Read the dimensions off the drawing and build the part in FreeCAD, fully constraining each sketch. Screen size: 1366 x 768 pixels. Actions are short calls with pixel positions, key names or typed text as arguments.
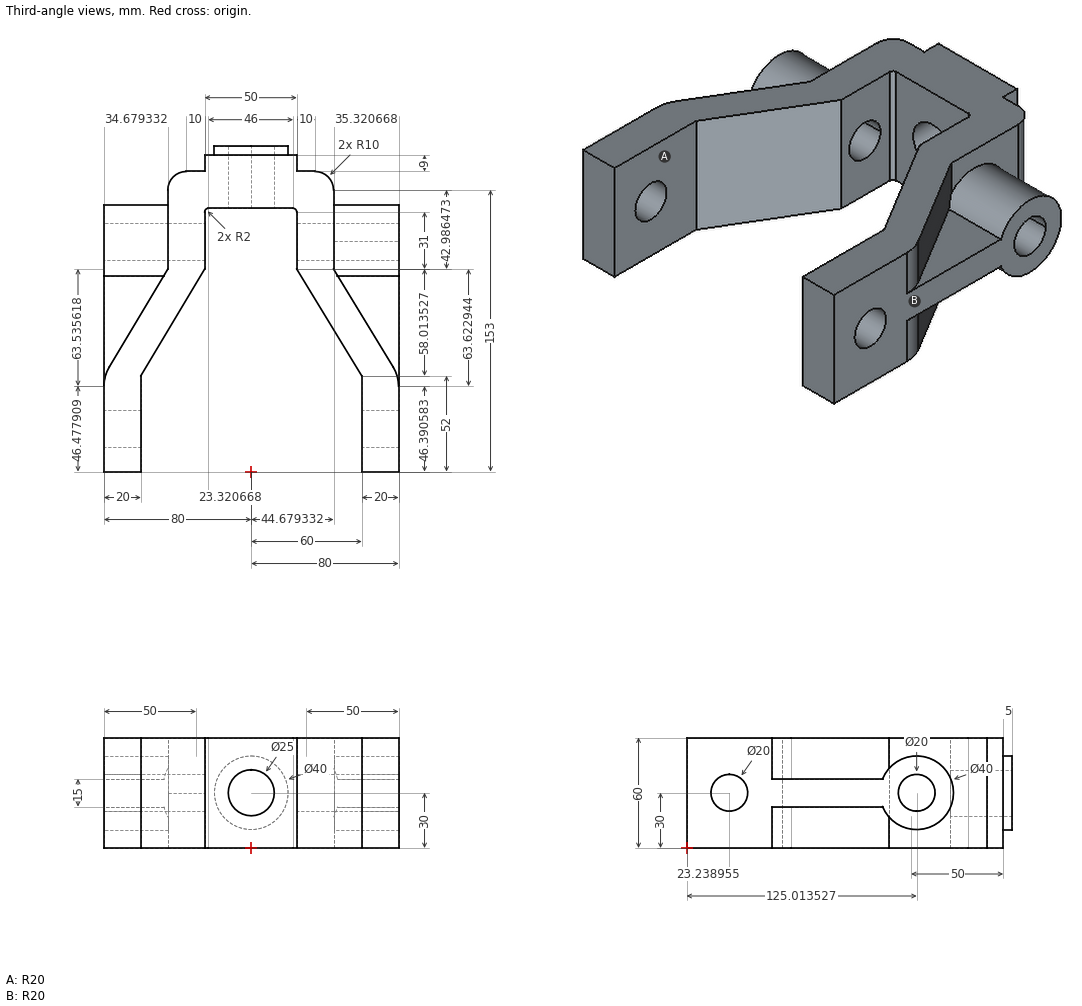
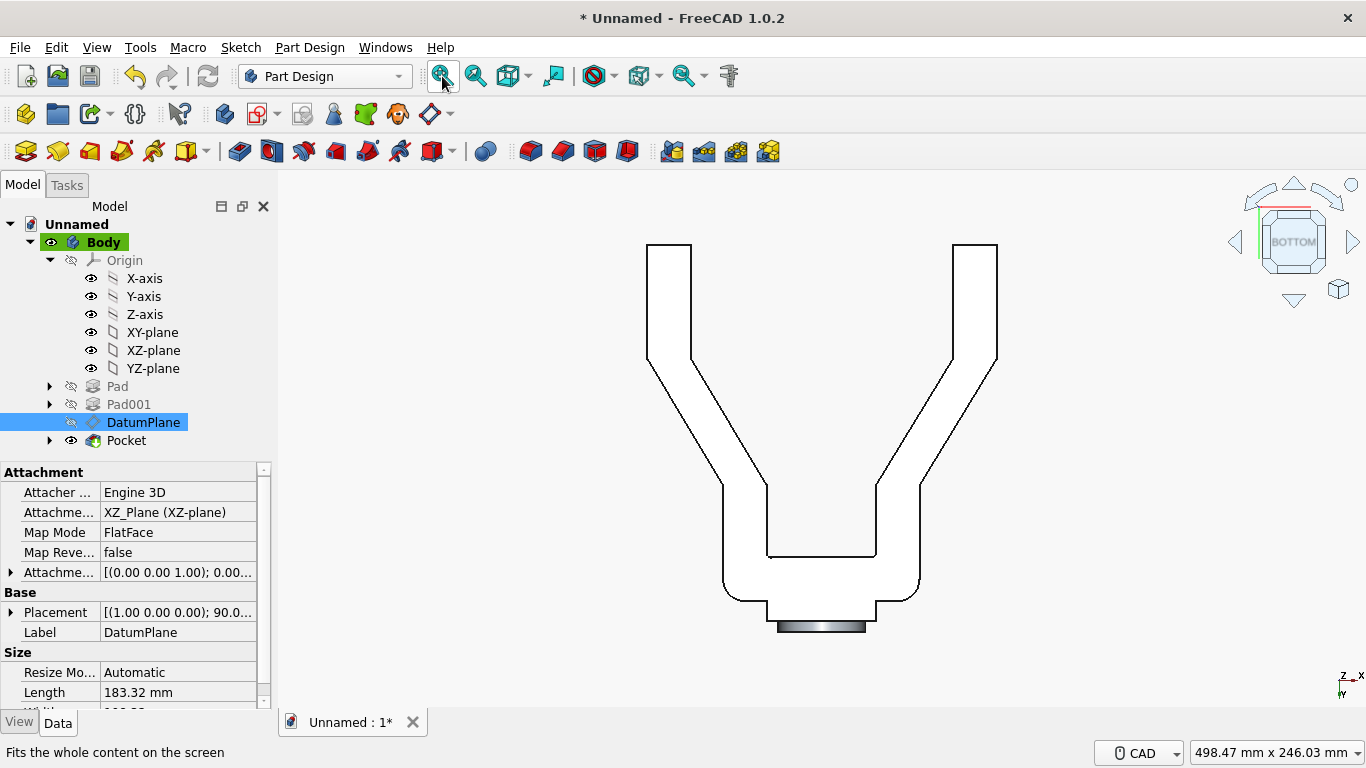
key(4)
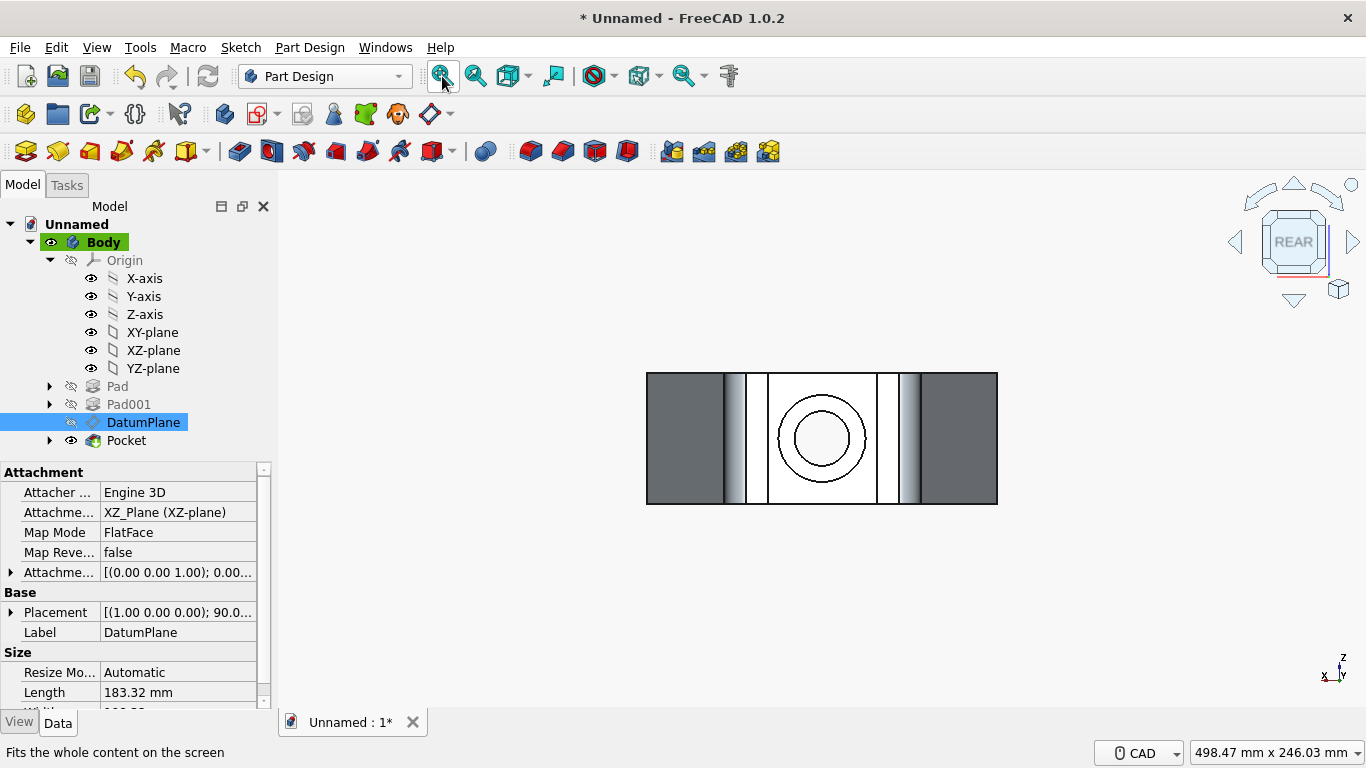
key(v)
key(f)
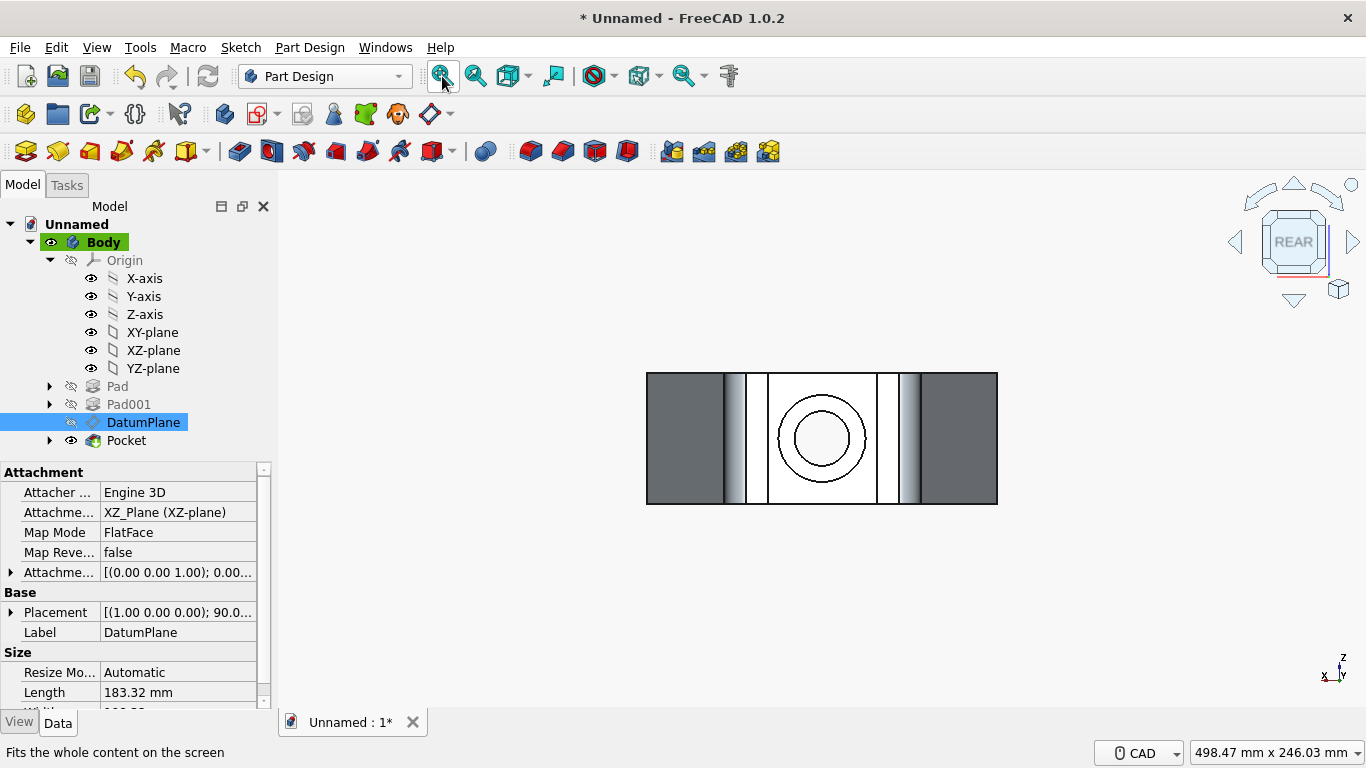
key(6)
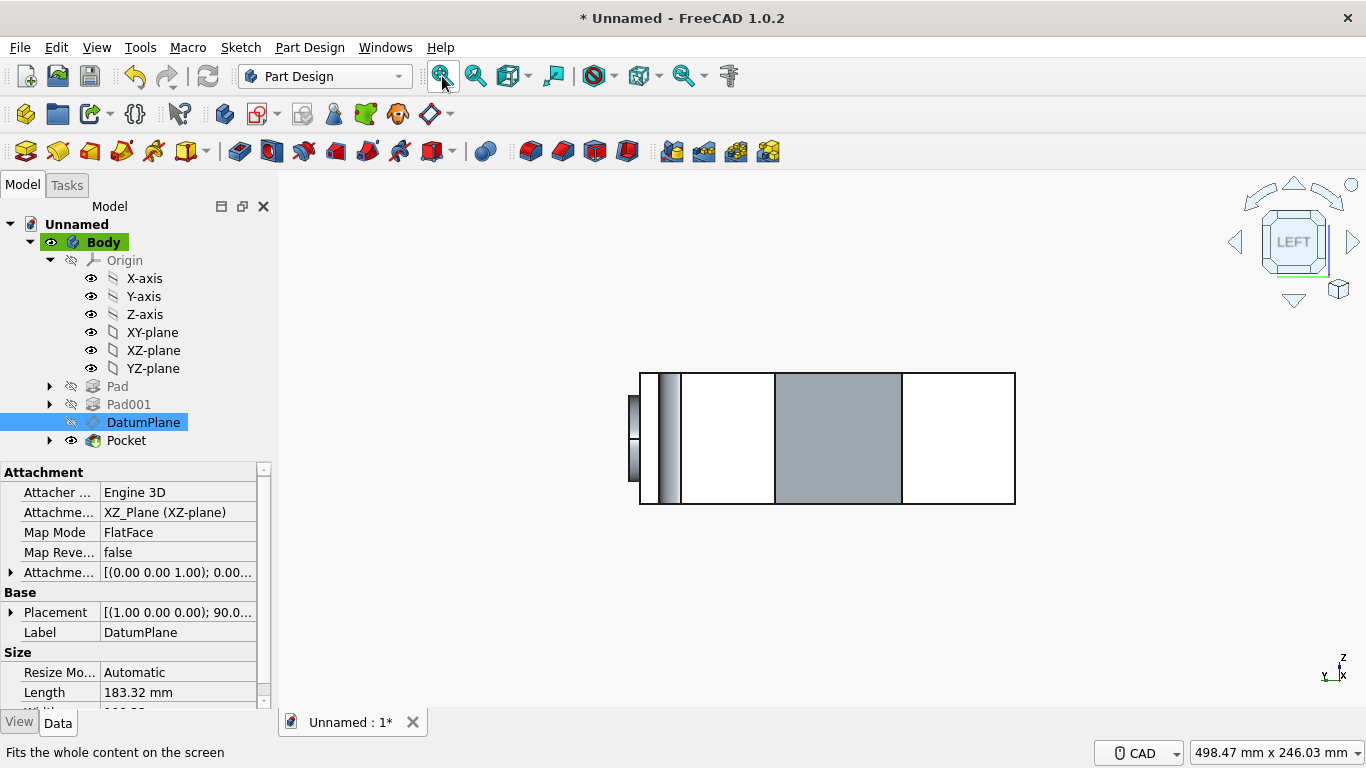
key(v)
key(f)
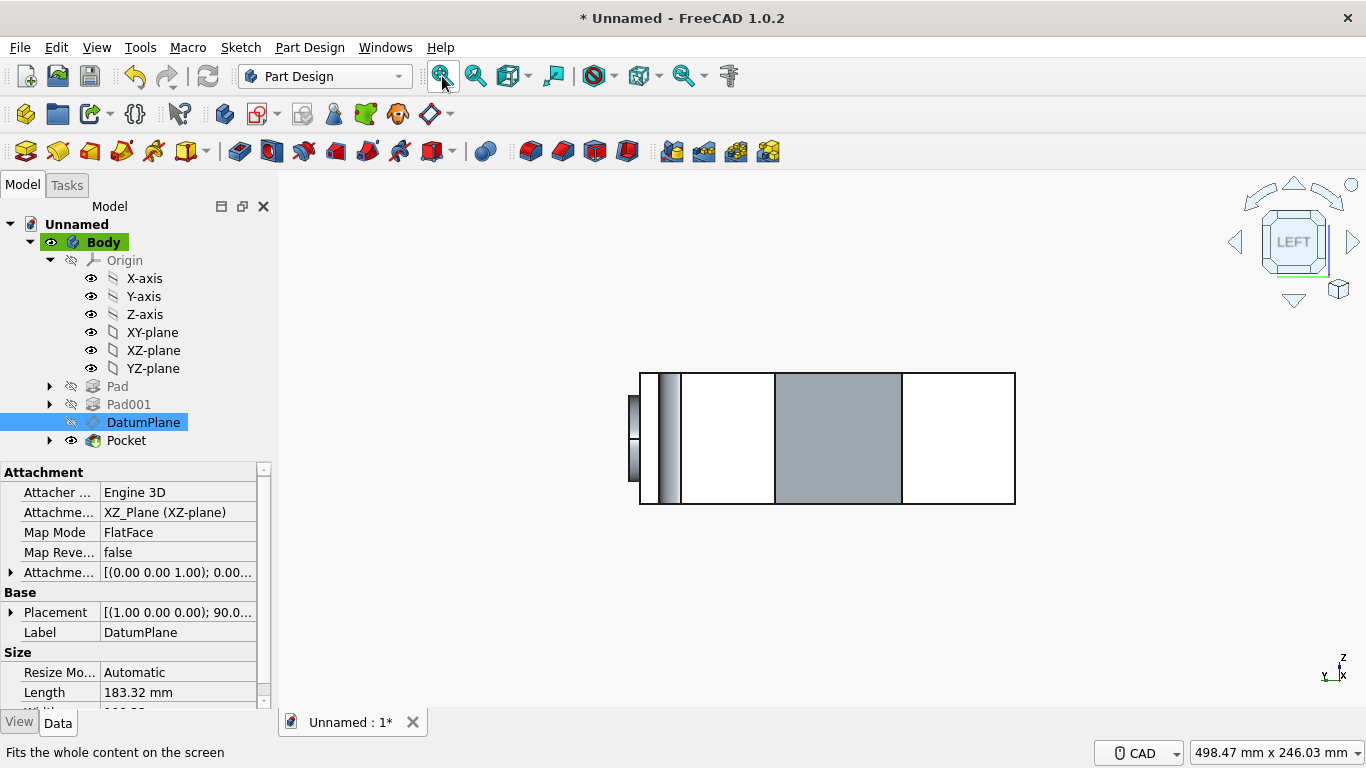
click(902, 437)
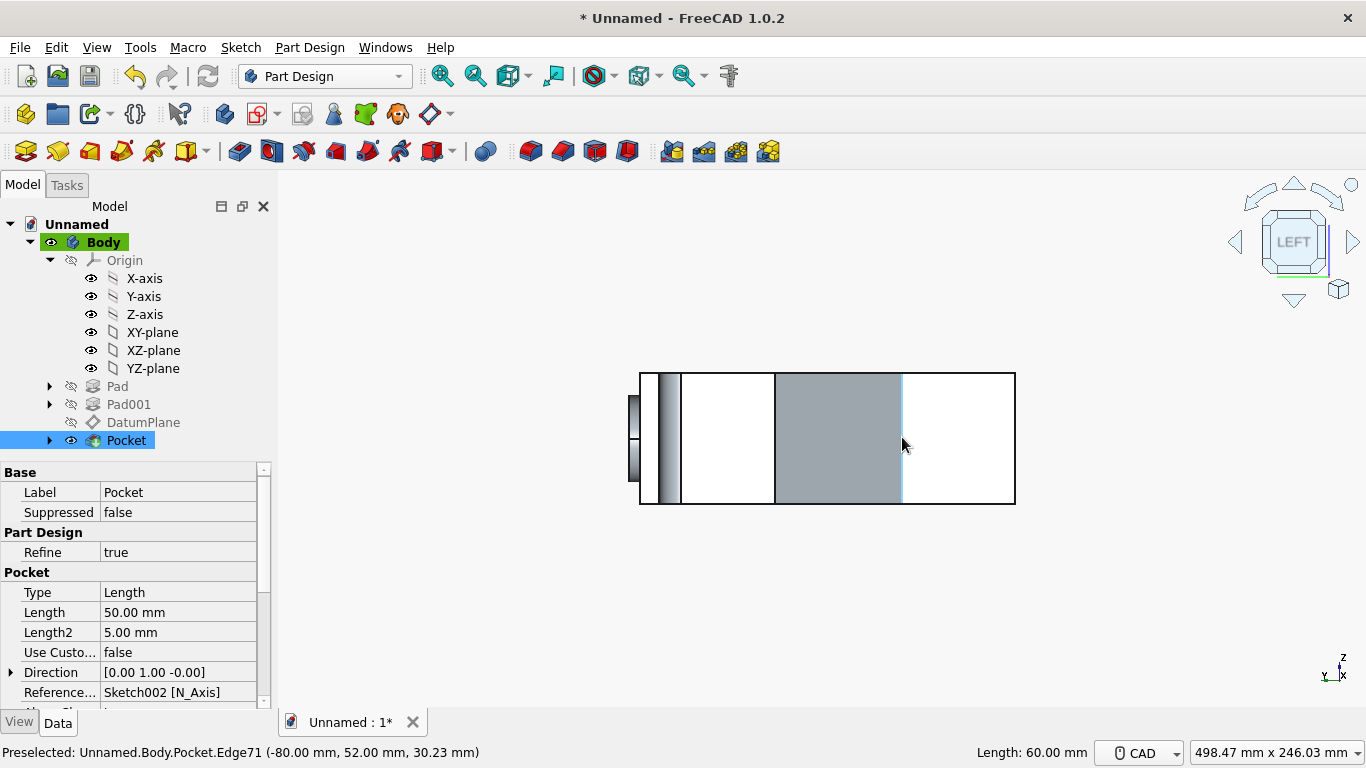
click(532, 152)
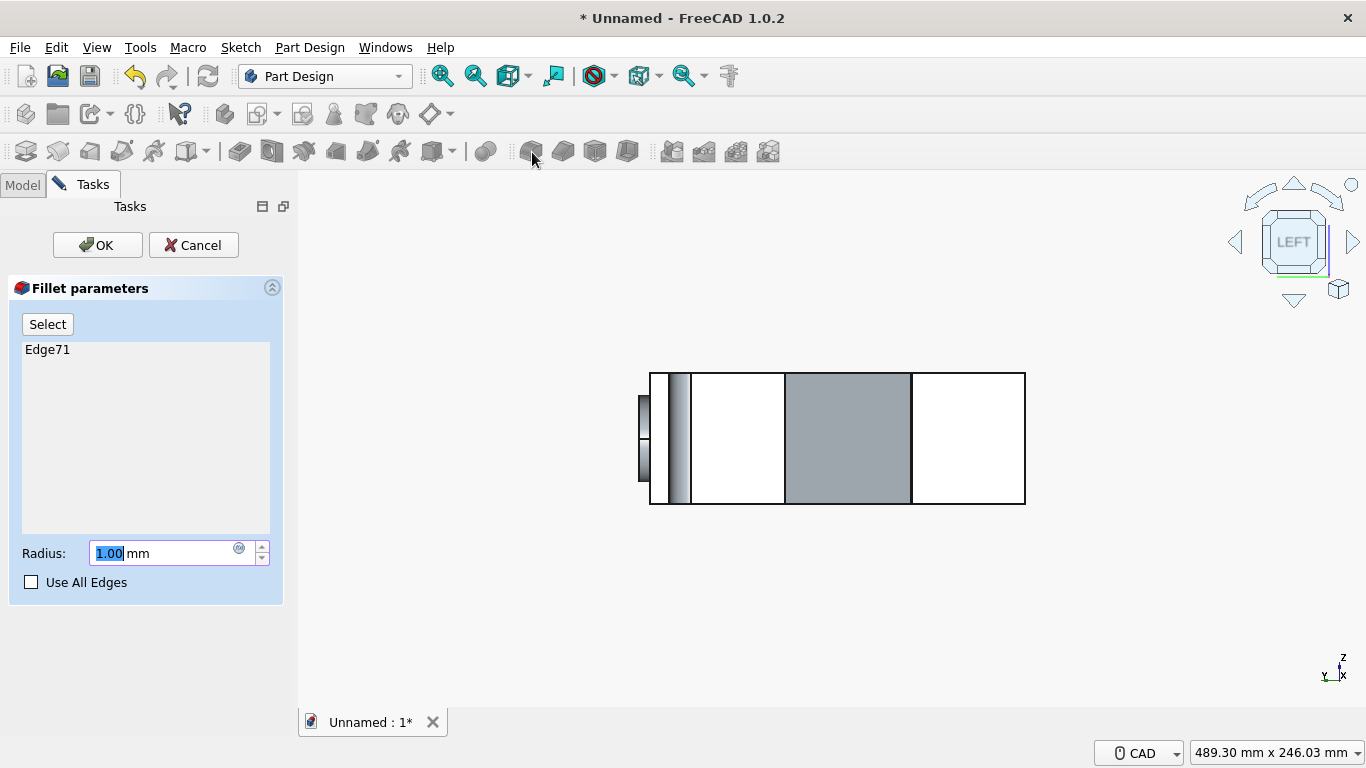
text(20)
key(Tab)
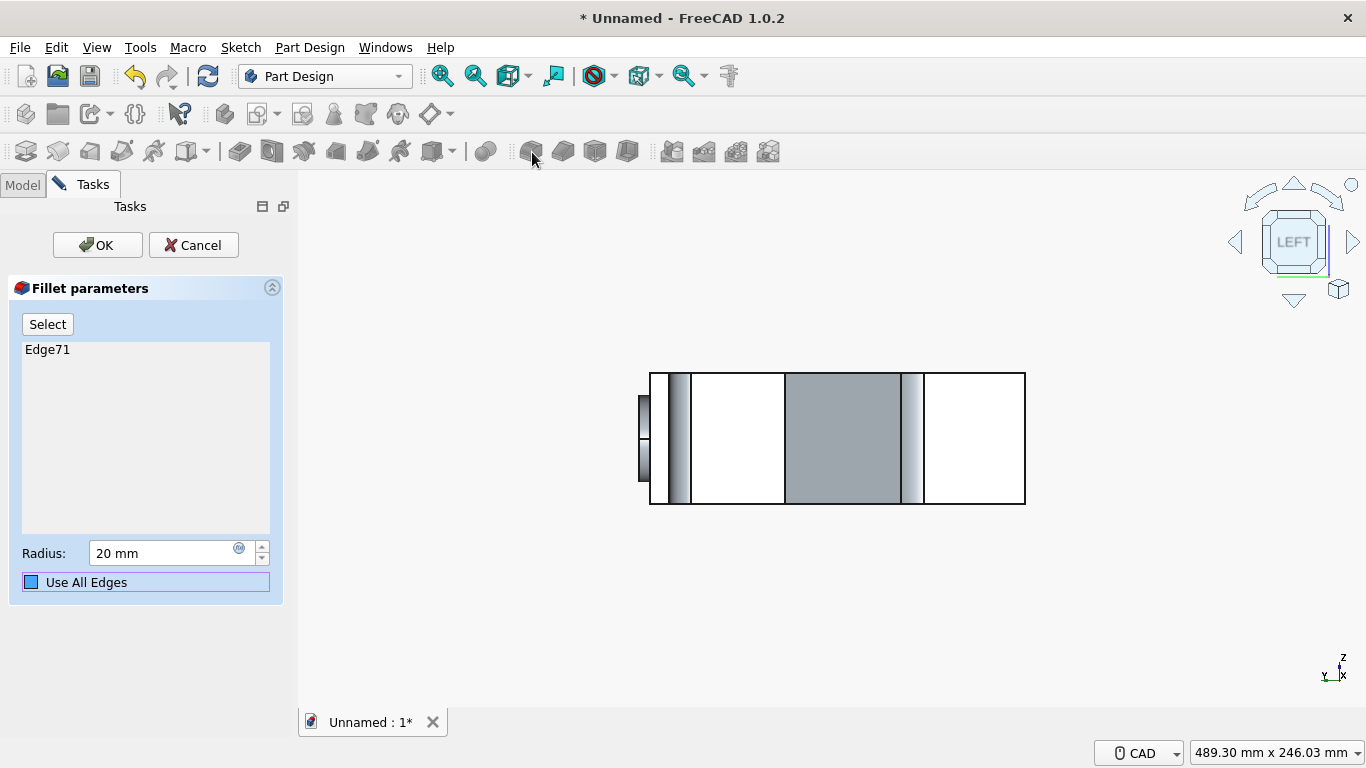
click(98, 245)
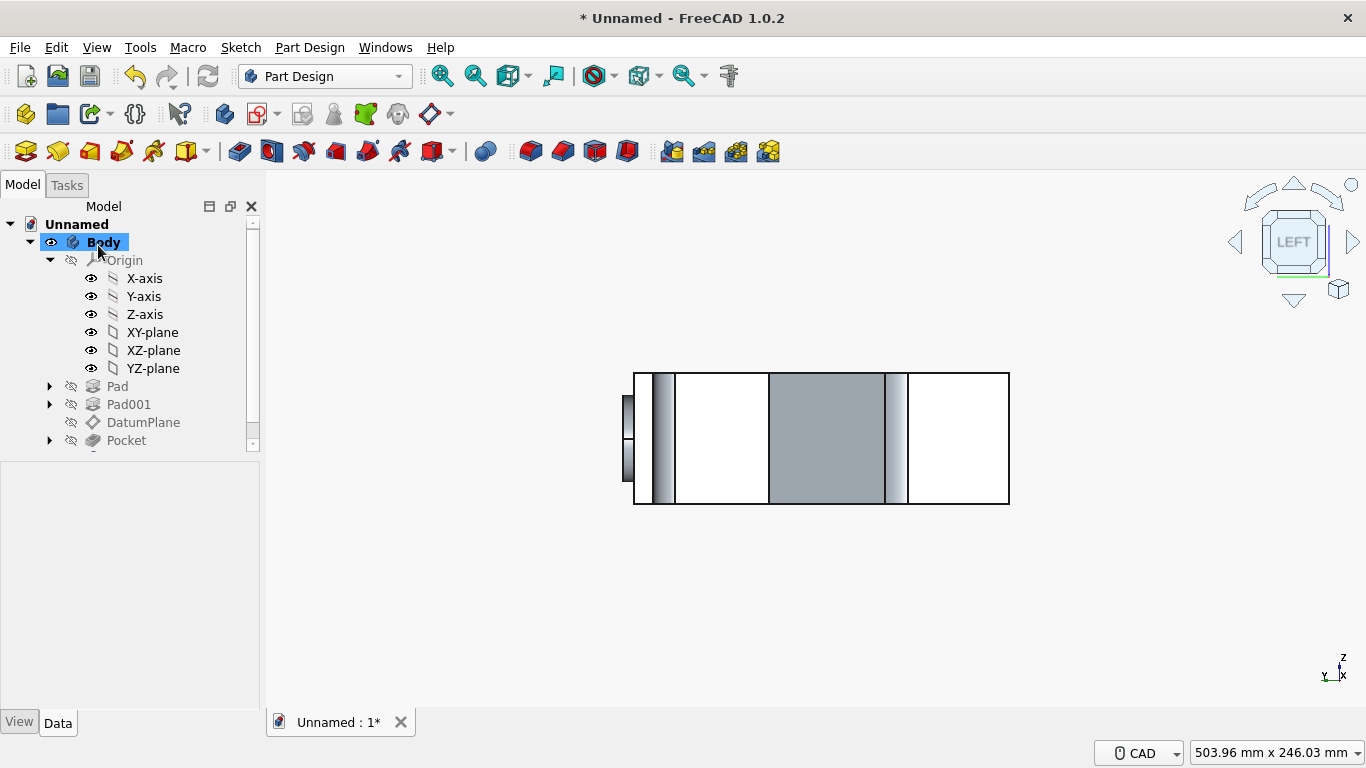
key(v)
key(f)